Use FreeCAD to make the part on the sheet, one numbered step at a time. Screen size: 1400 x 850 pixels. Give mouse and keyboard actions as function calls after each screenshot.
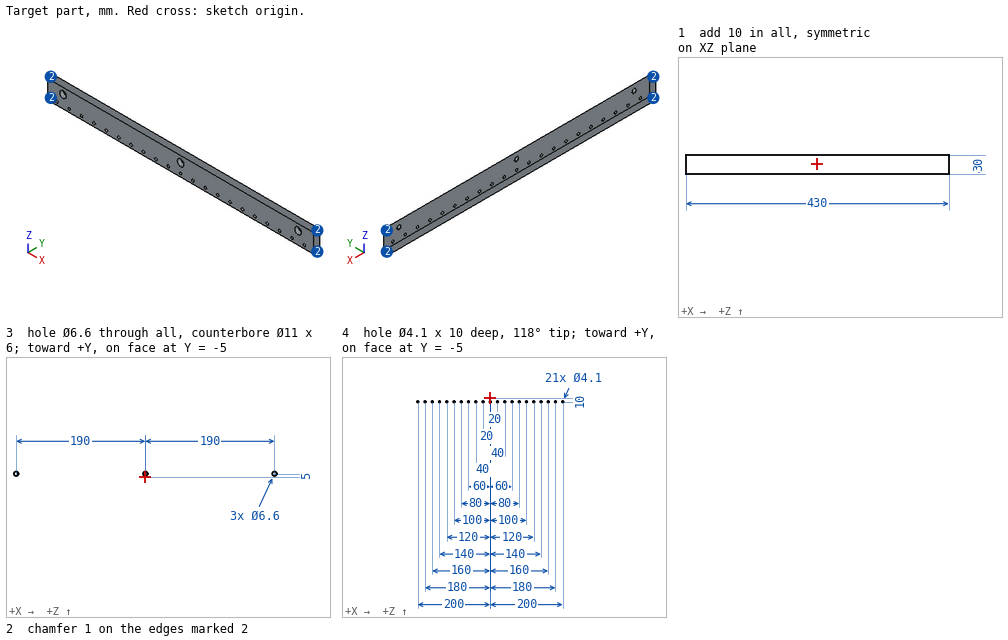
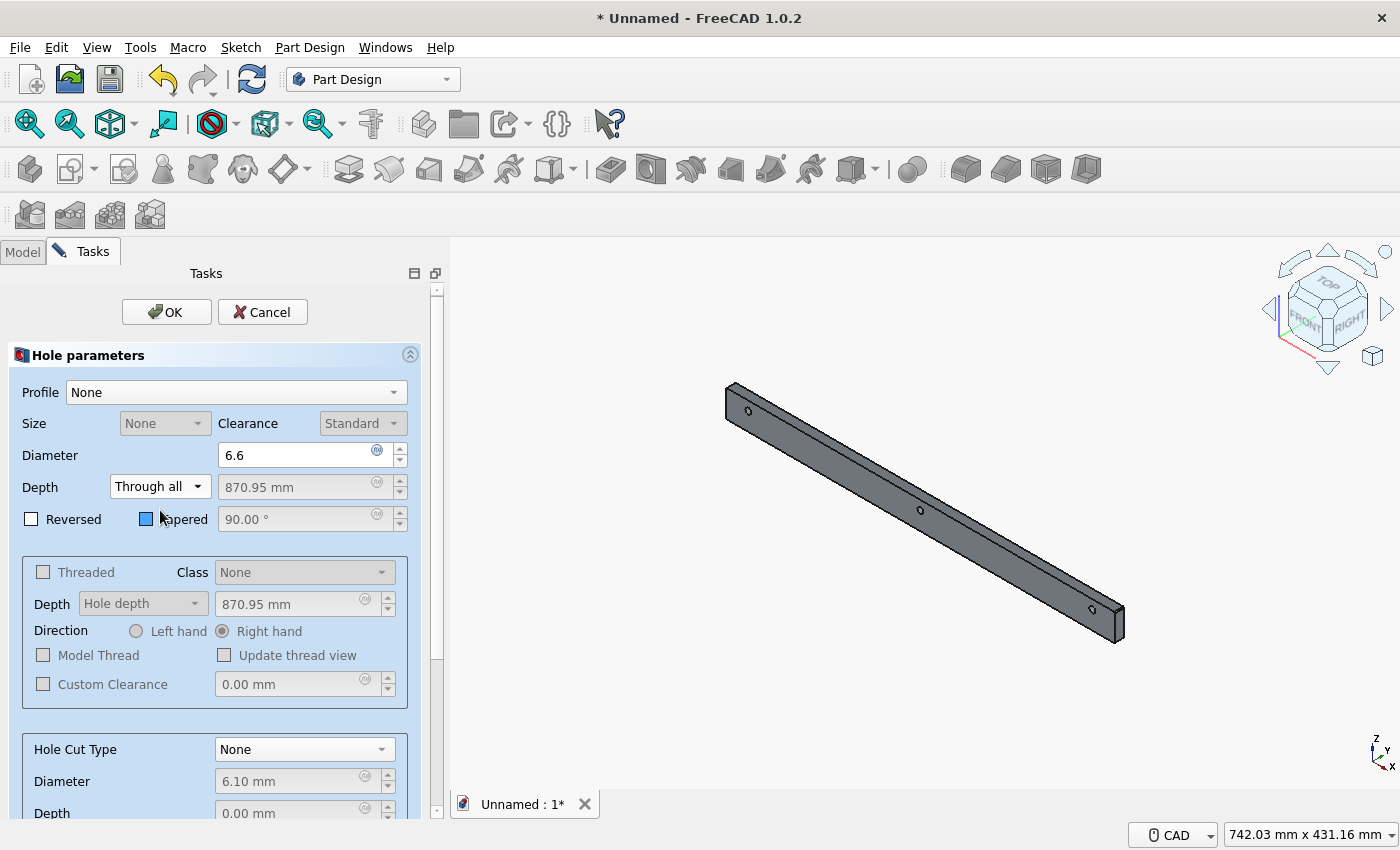
click(306, 750)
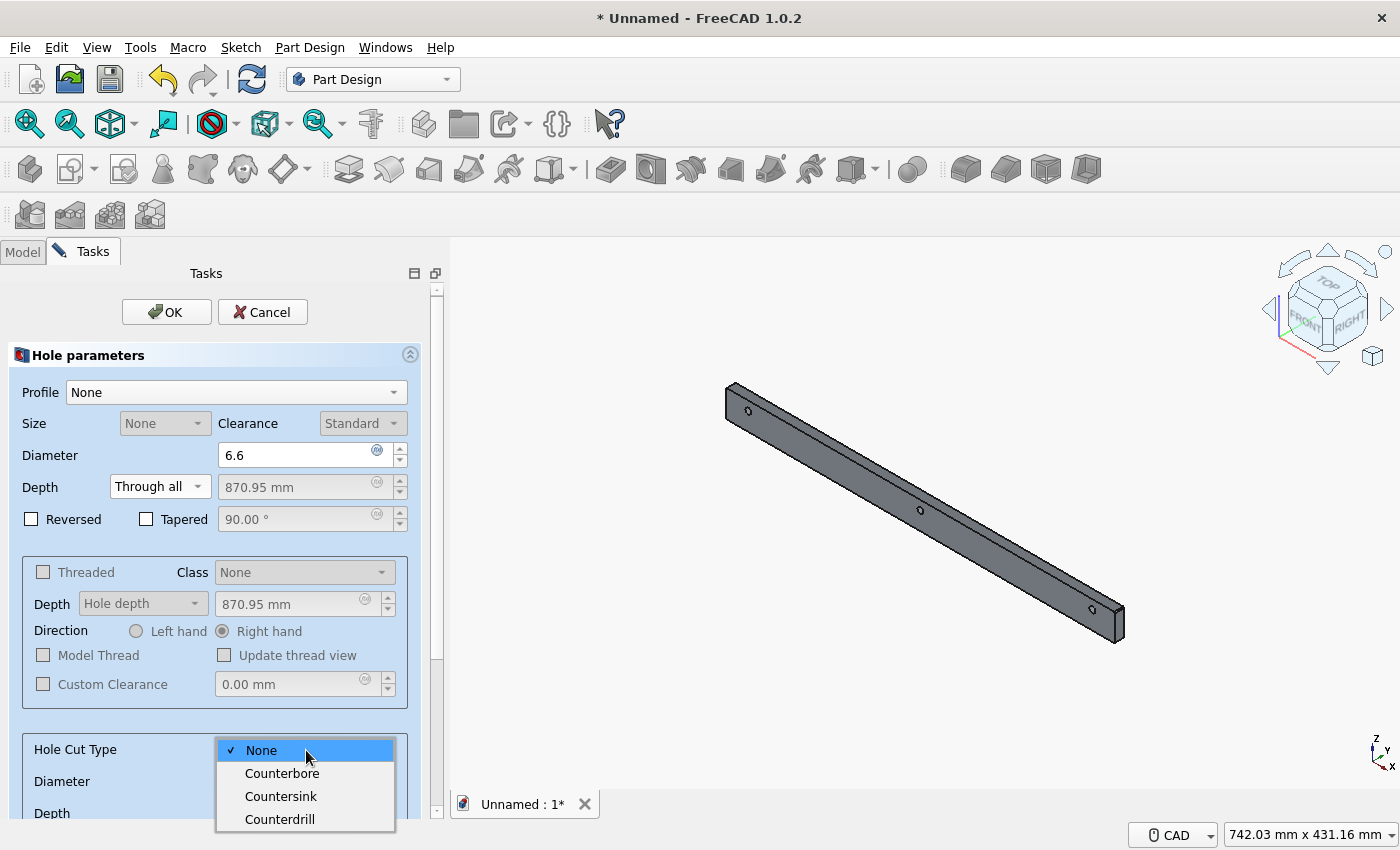
click(304, 774)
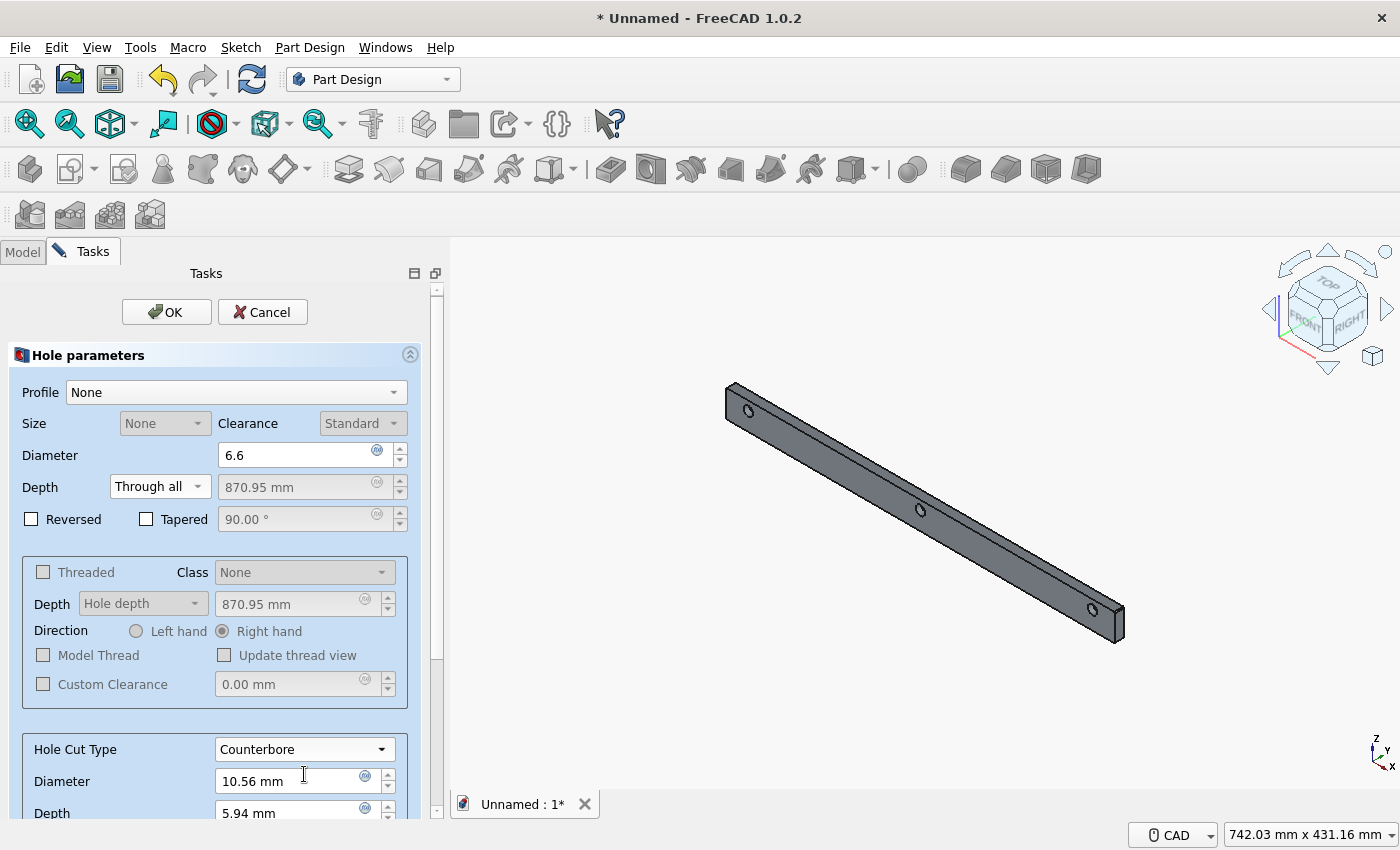
triple_click(298, 781)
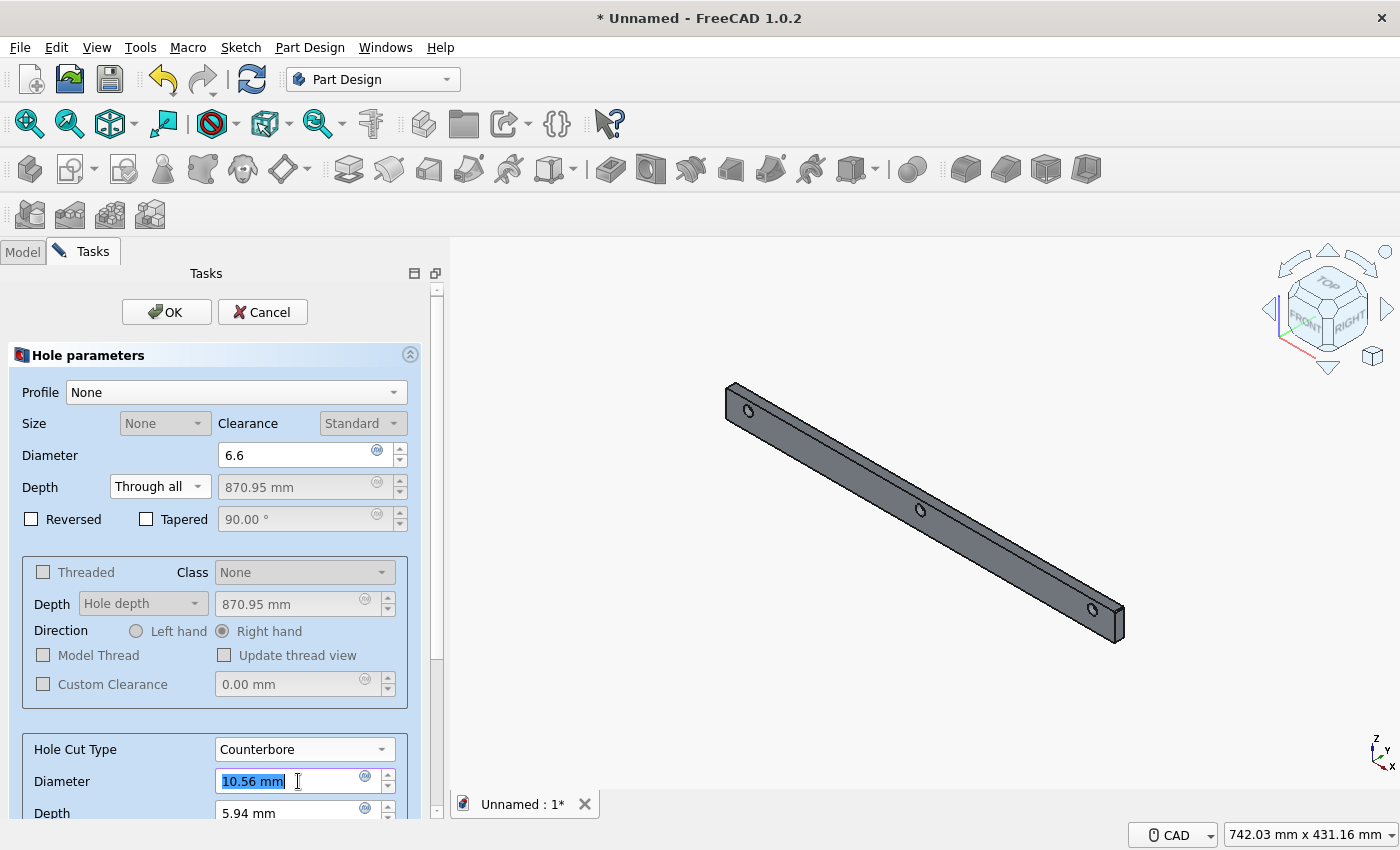
text(11)
key(Tab)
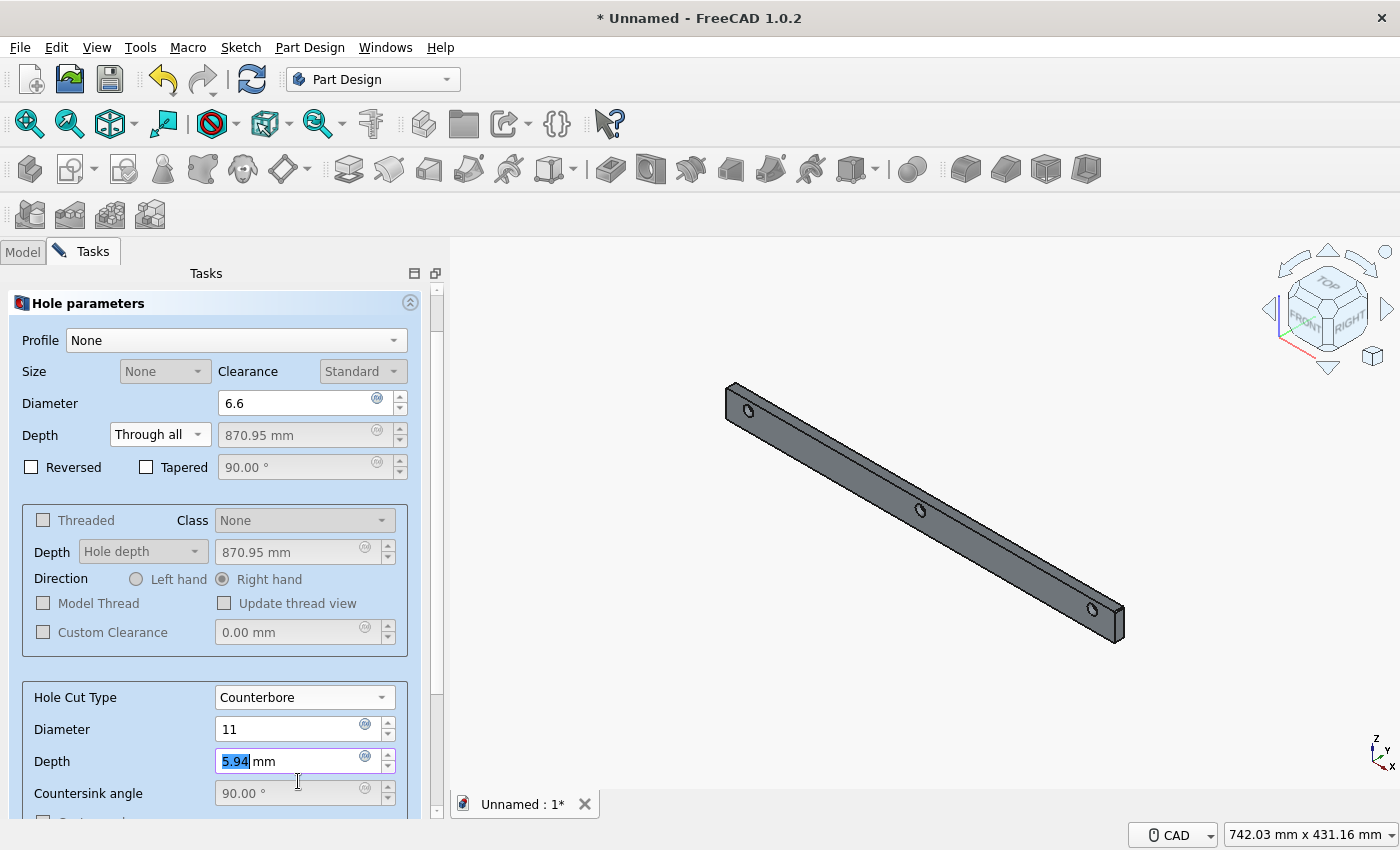
text(6)
key(Tab)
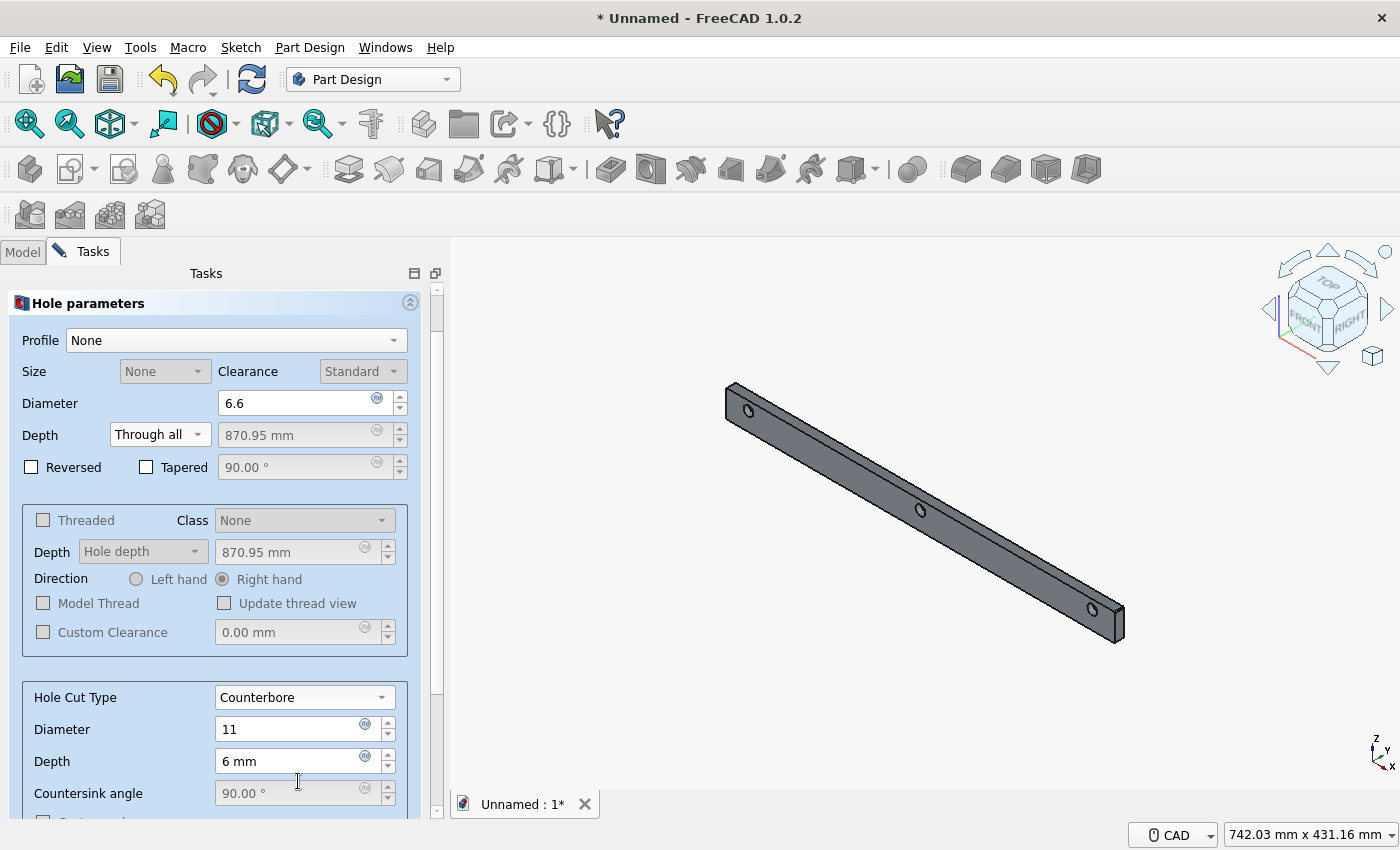
scroll(437, 550, up, 2)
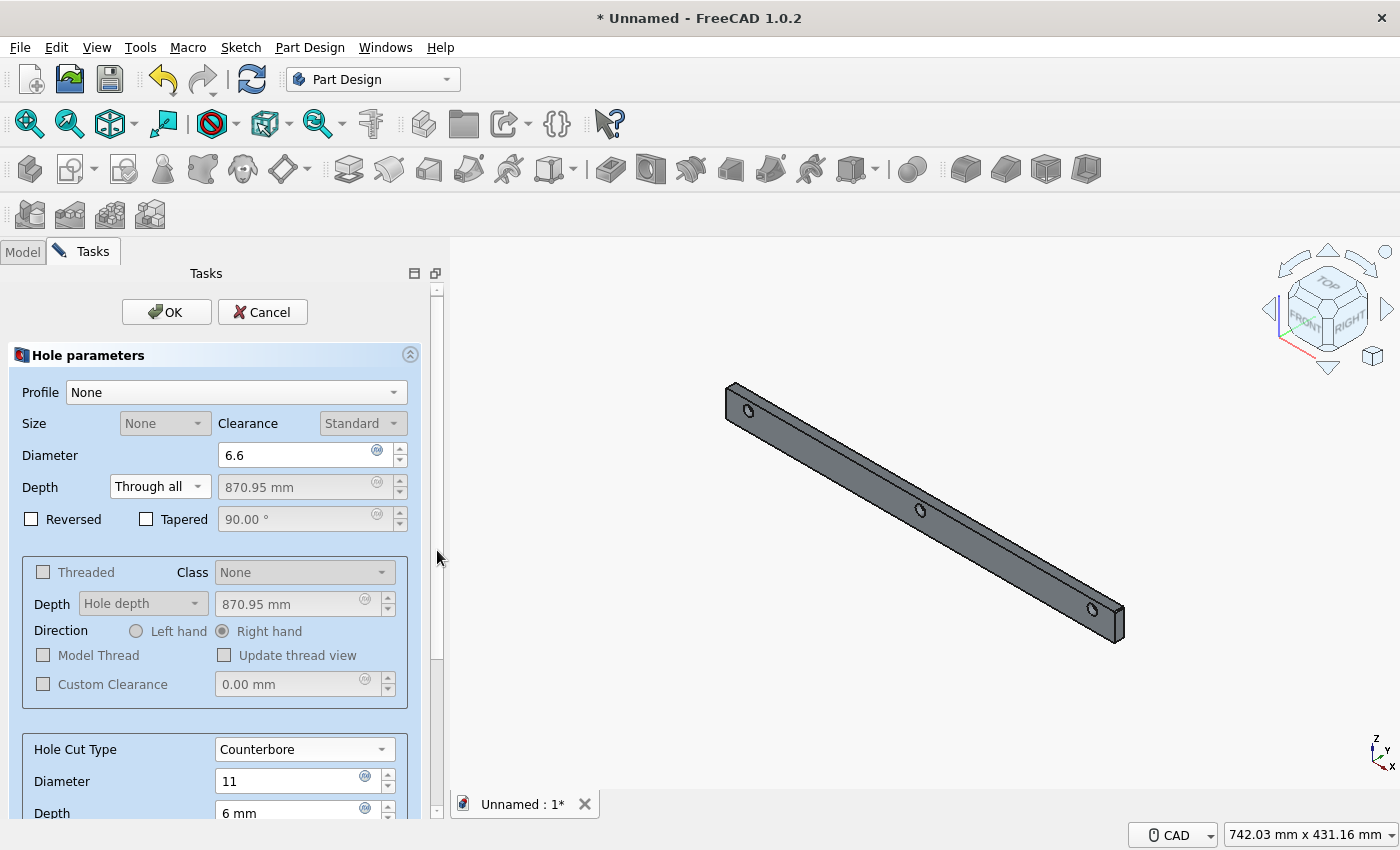
click(167, 312)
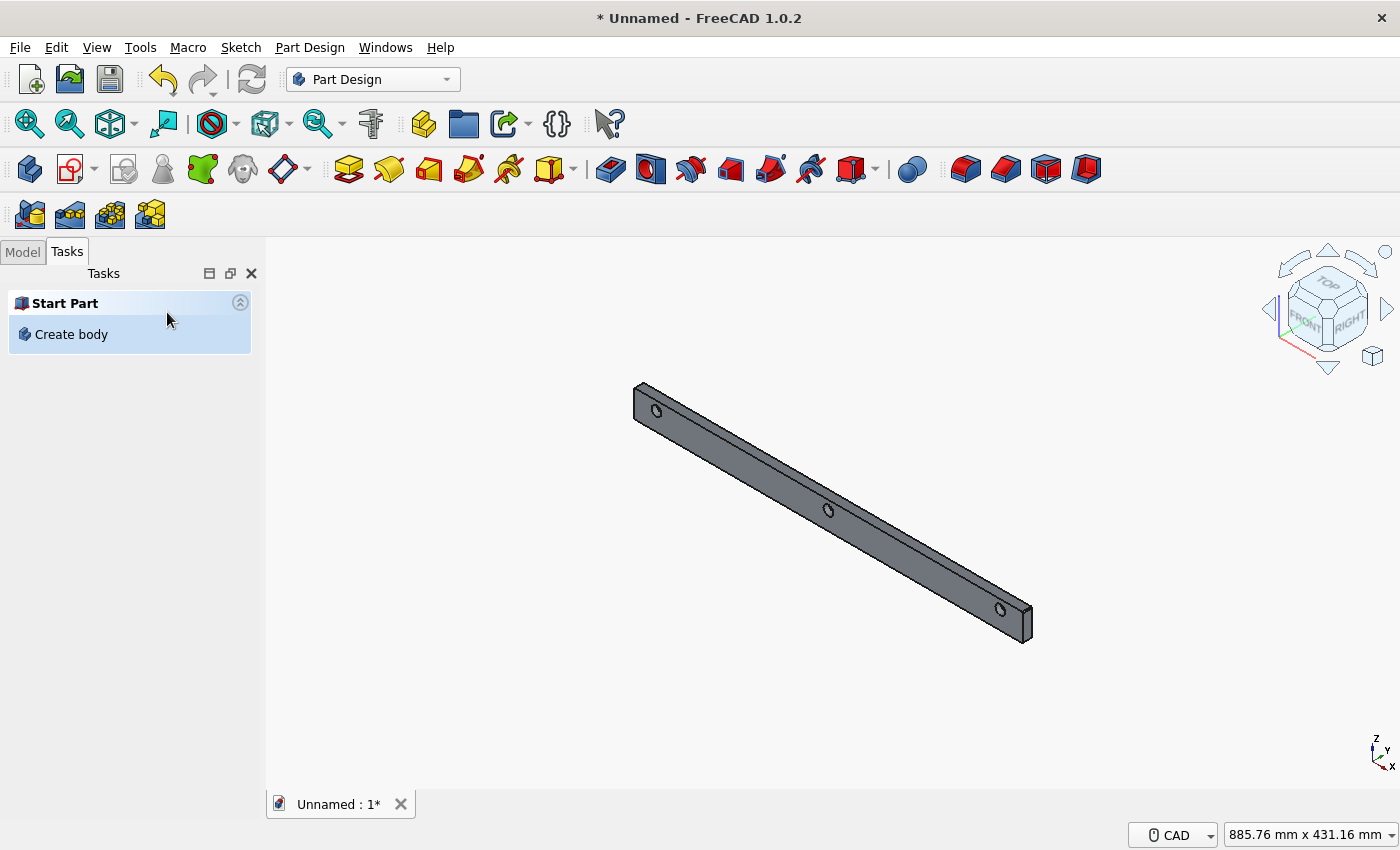
click(940, 579)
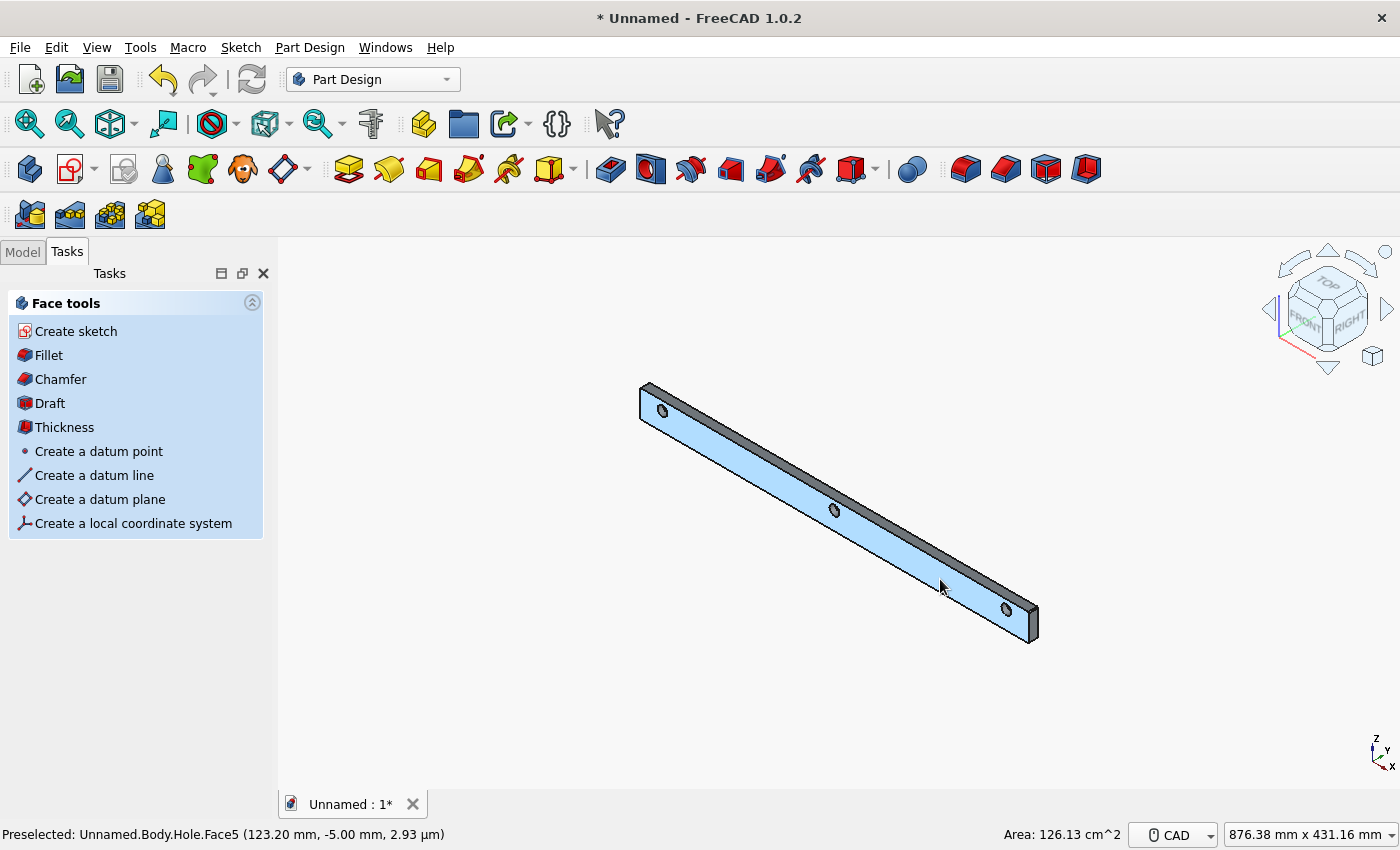
click(70, 170)